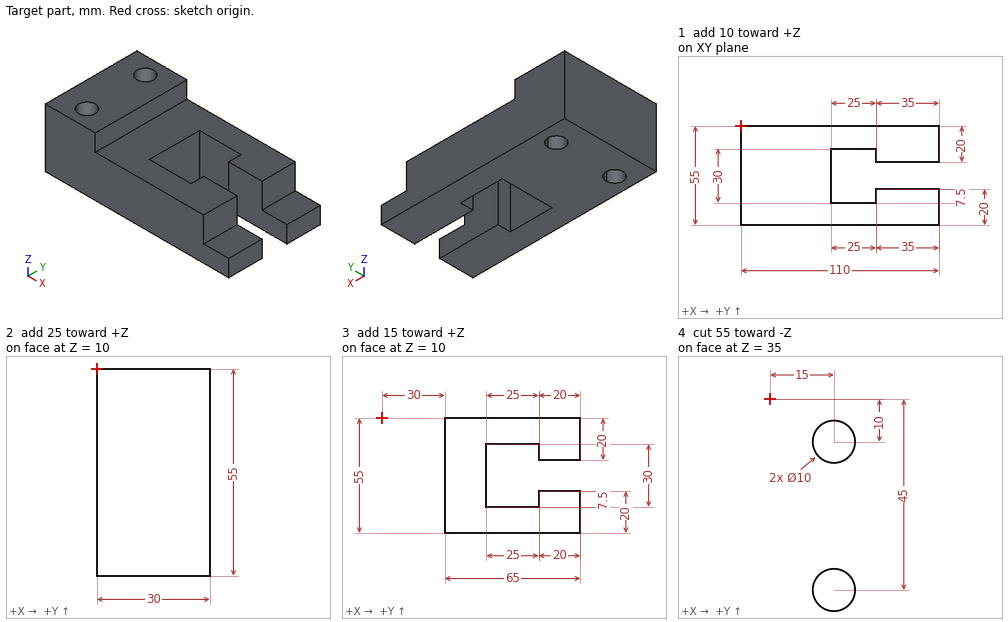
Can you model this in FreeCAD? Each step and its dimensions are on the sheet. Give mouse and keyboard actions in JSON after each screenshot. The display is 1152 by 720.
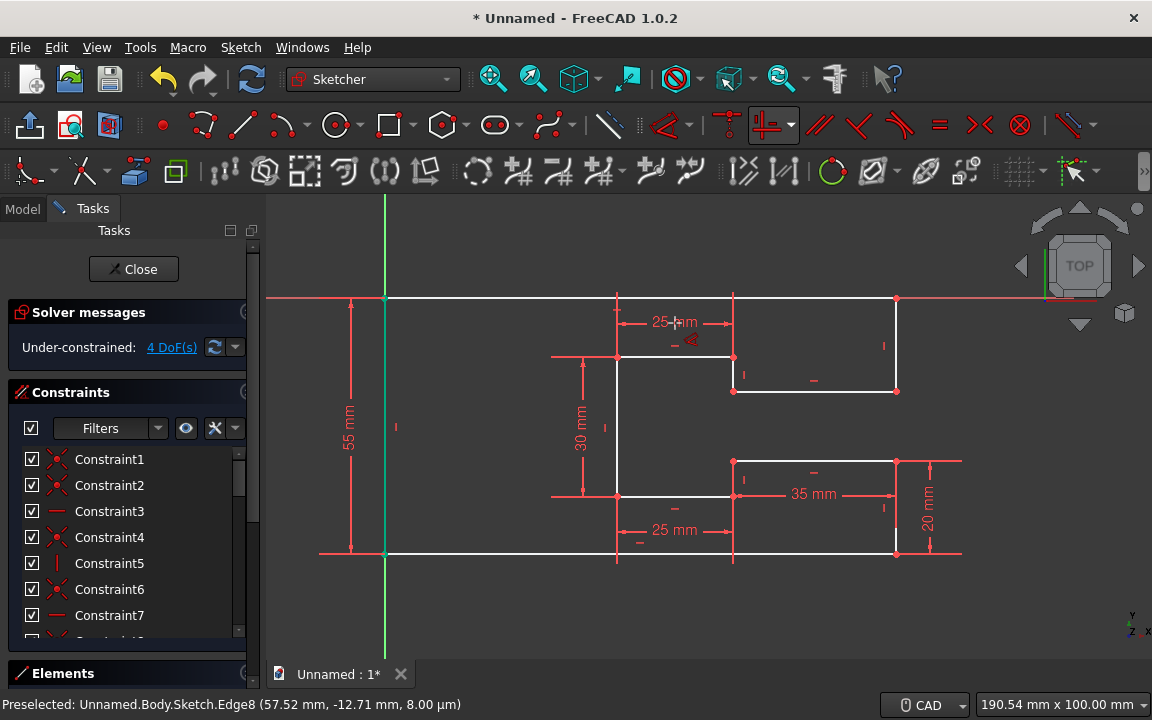
{"action": "left_click", "coordinate": [782, 392]}
{"action": "left_click", "coordinate": [815, 358]}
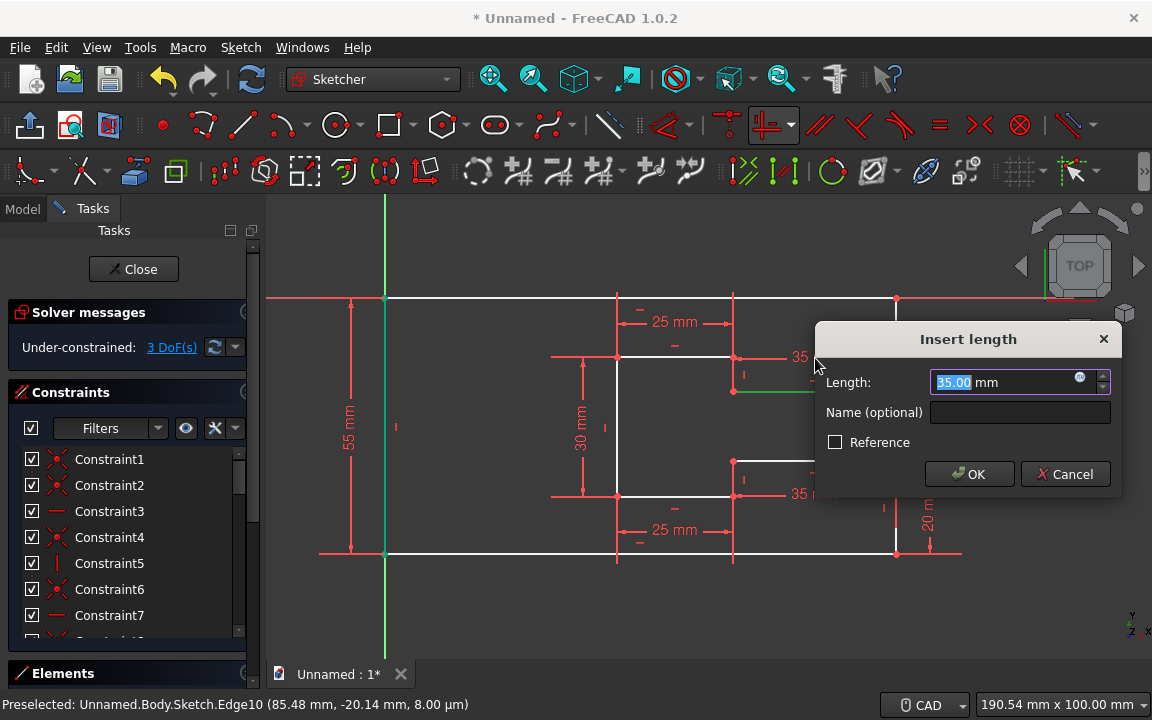
{"action": "type", "text": "35"}
{"action": "key", "text": "Return"}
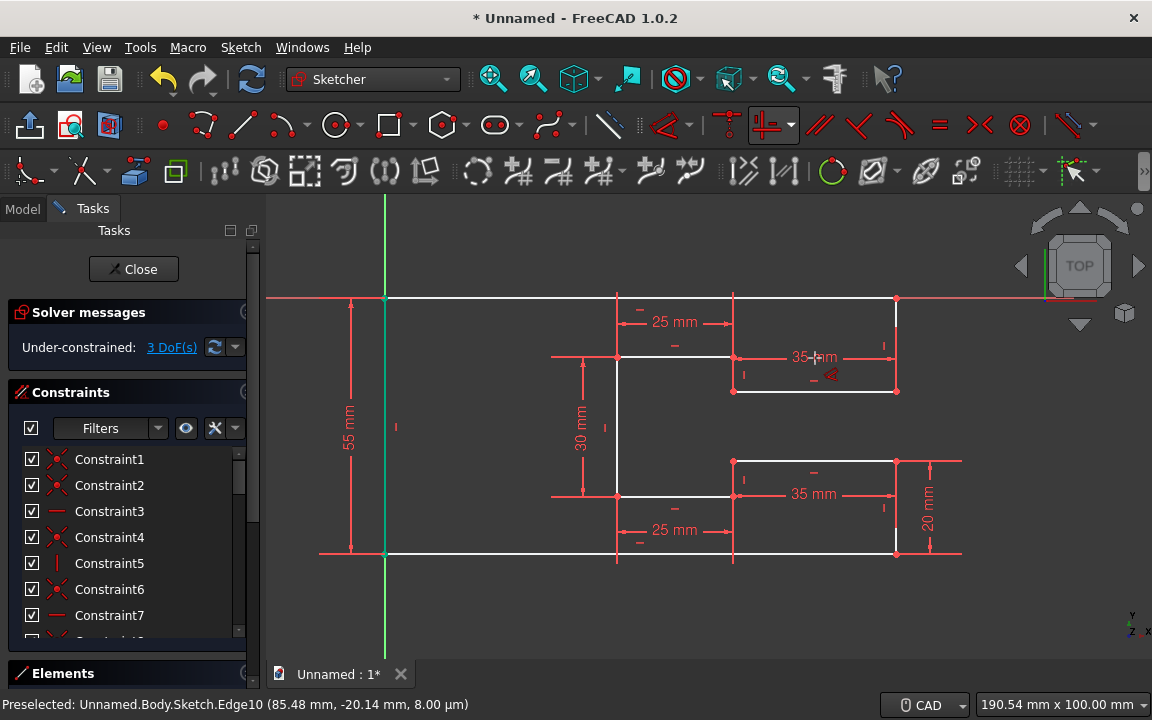
{"action": "left_click", "coordinate": [896, 364]}
{"action": "left_click", "coordinate": [930, 345]}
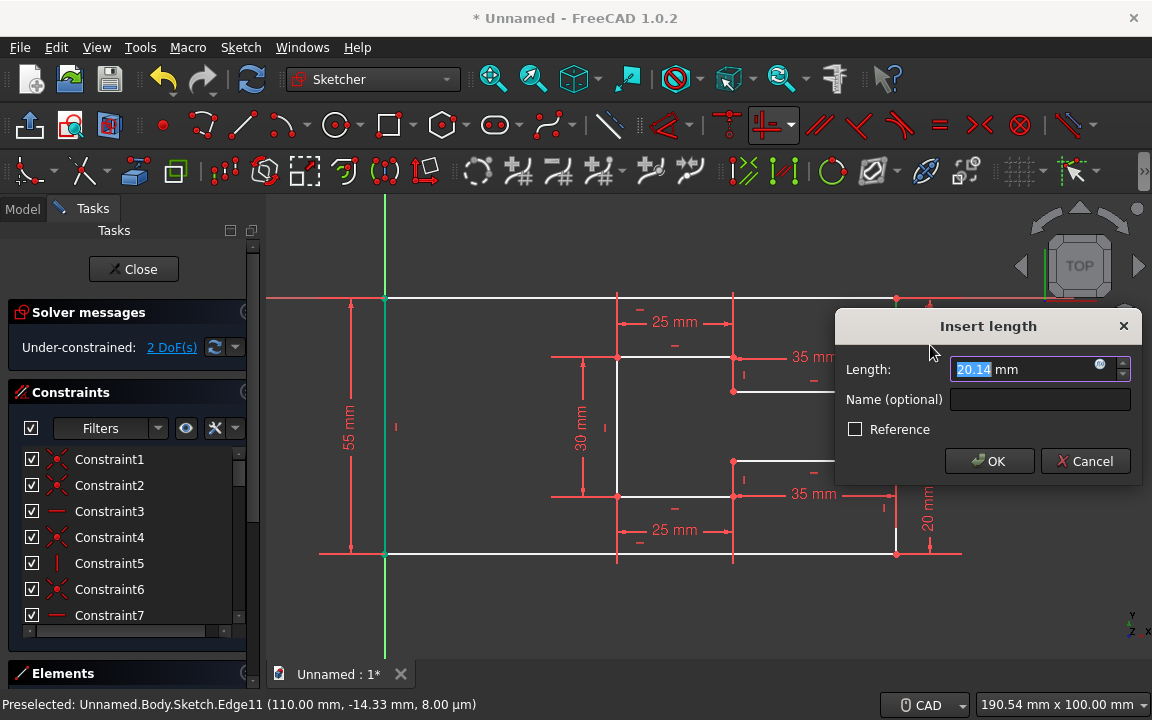
{"action": "type", "text": "20"}
{"action": "key", "text": "Return"}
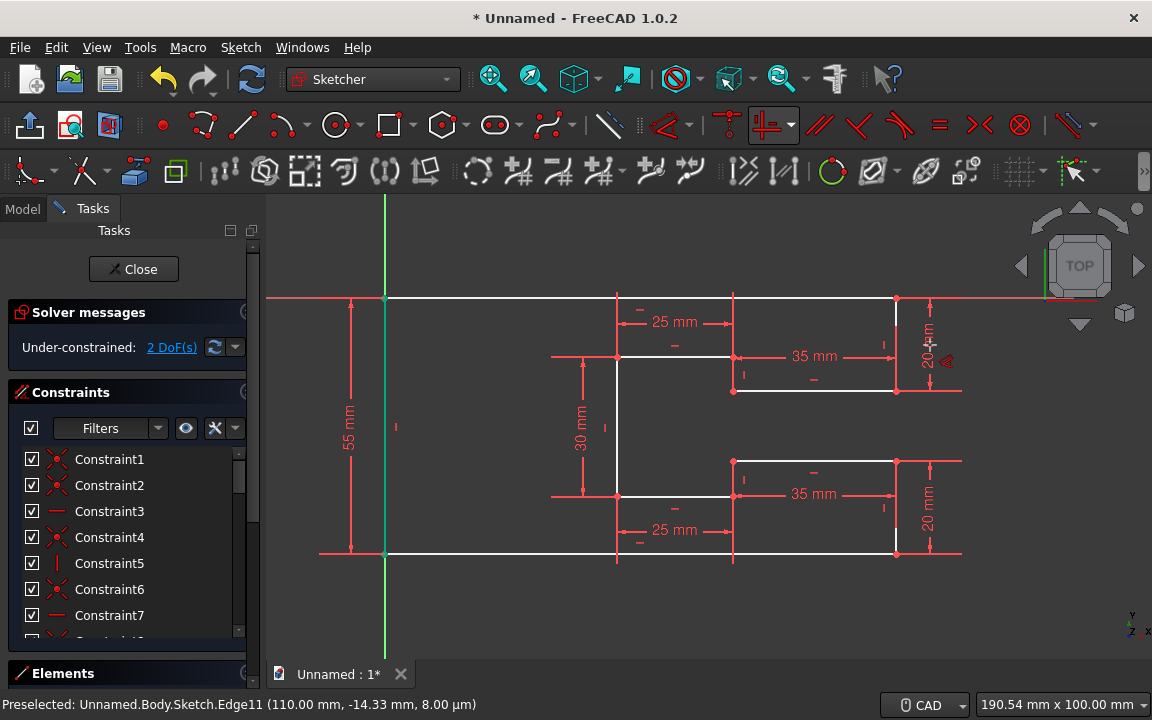
{"action": "left_click", "coordinate": [538, 554]}
{"action": "left_click", "coordinate": [640, 588]}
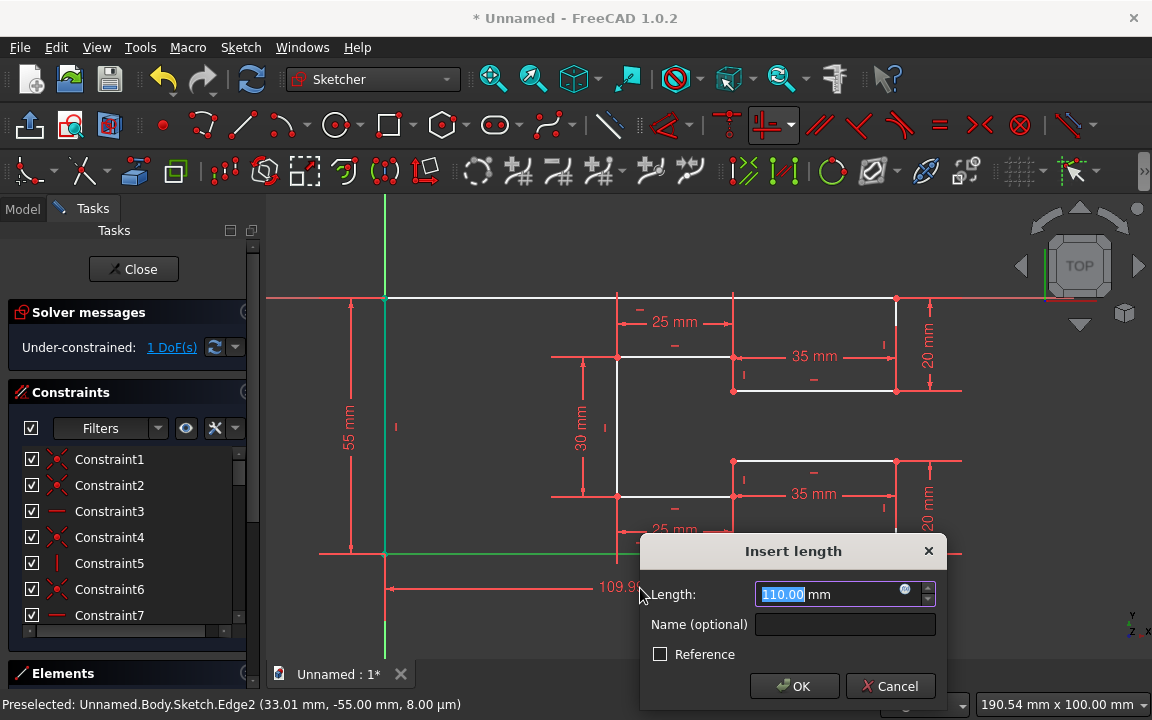
{"action": "type", "text": "110"}
{"action": "key", "text": "Return"}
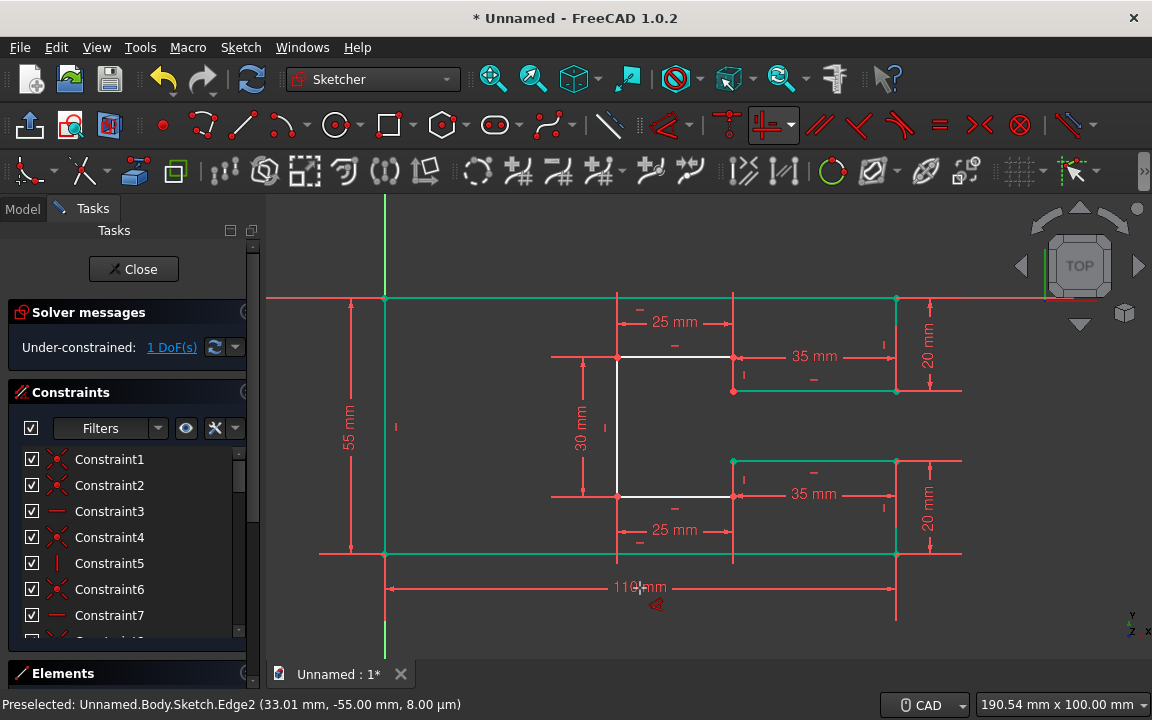
{"action": "scroll", "coordinate": [733, 472], "scroll_direction": "up", "scroll_amount": 2}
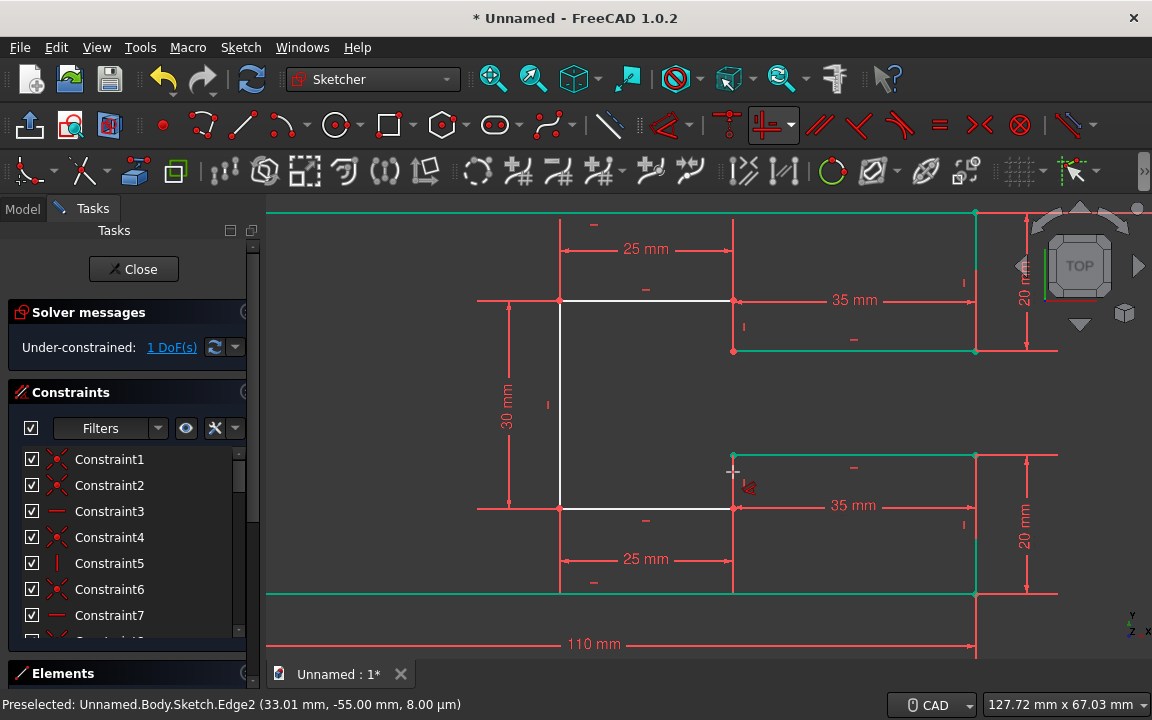
{"action": "left_click", "coordinate": [733, 471]}
{"action": "left_click", "coordinate": [767, 482]}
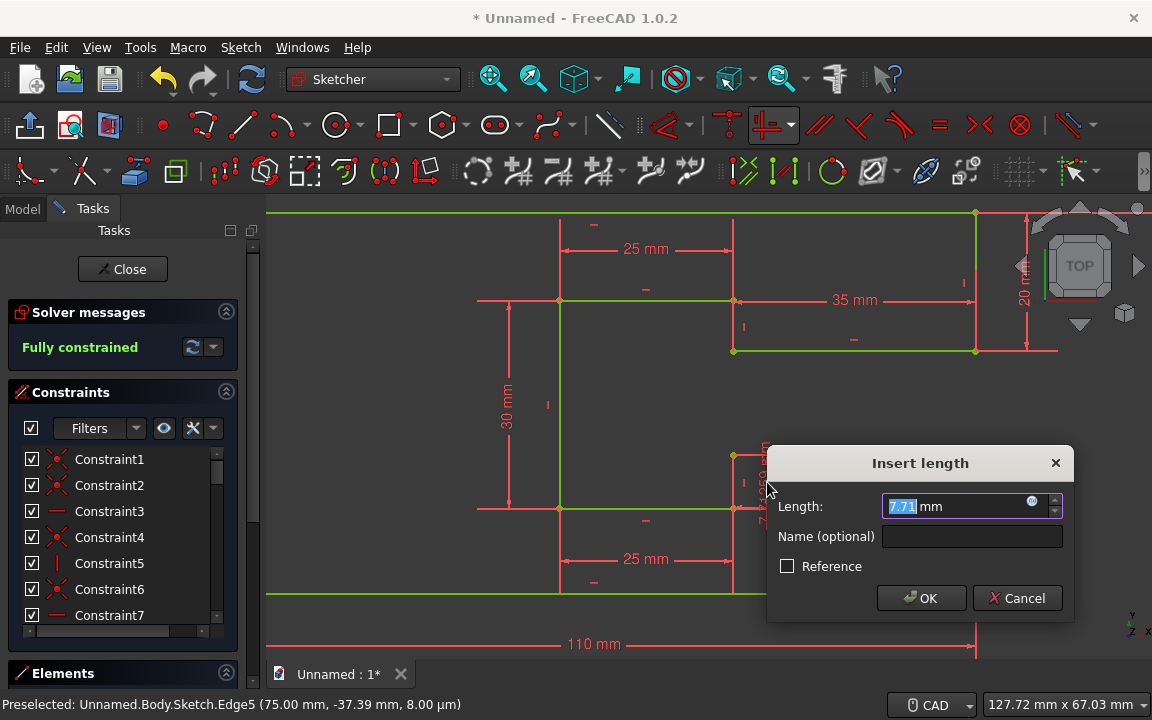
{"action": "type", "text": "7.5"}
{"action": "key", "text": "Return"}
{"action": "key", "text": "Escape"}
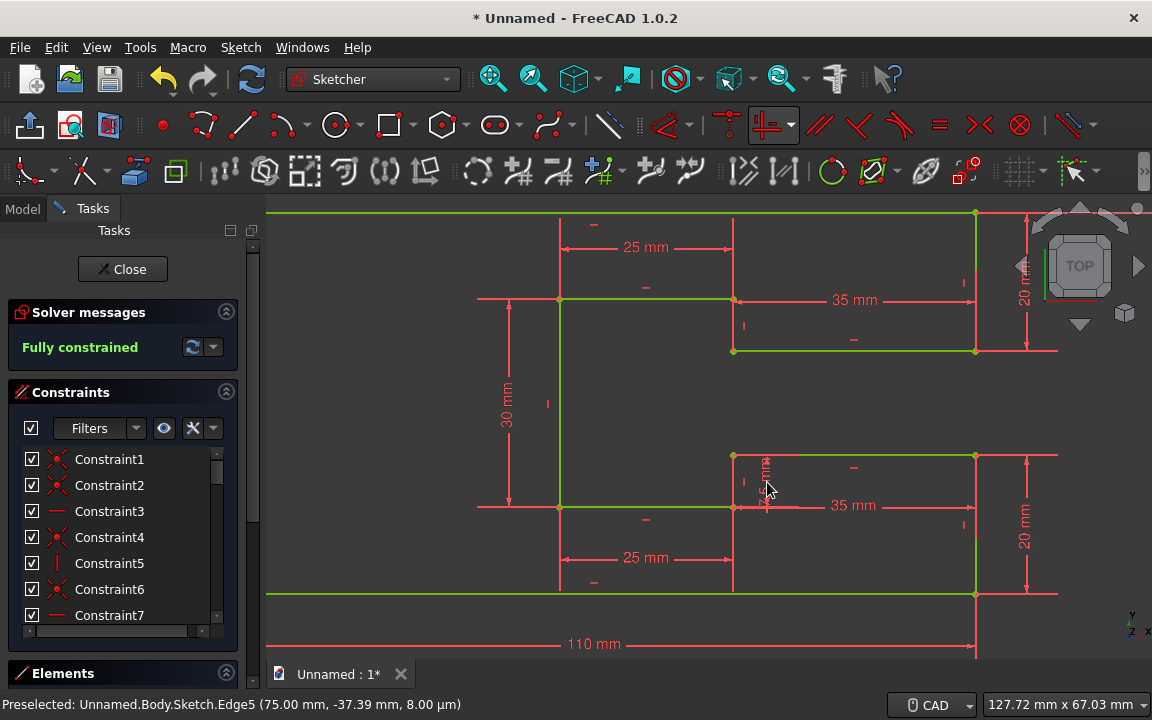
{"action": "left_click", "coordinate": [123, 269]}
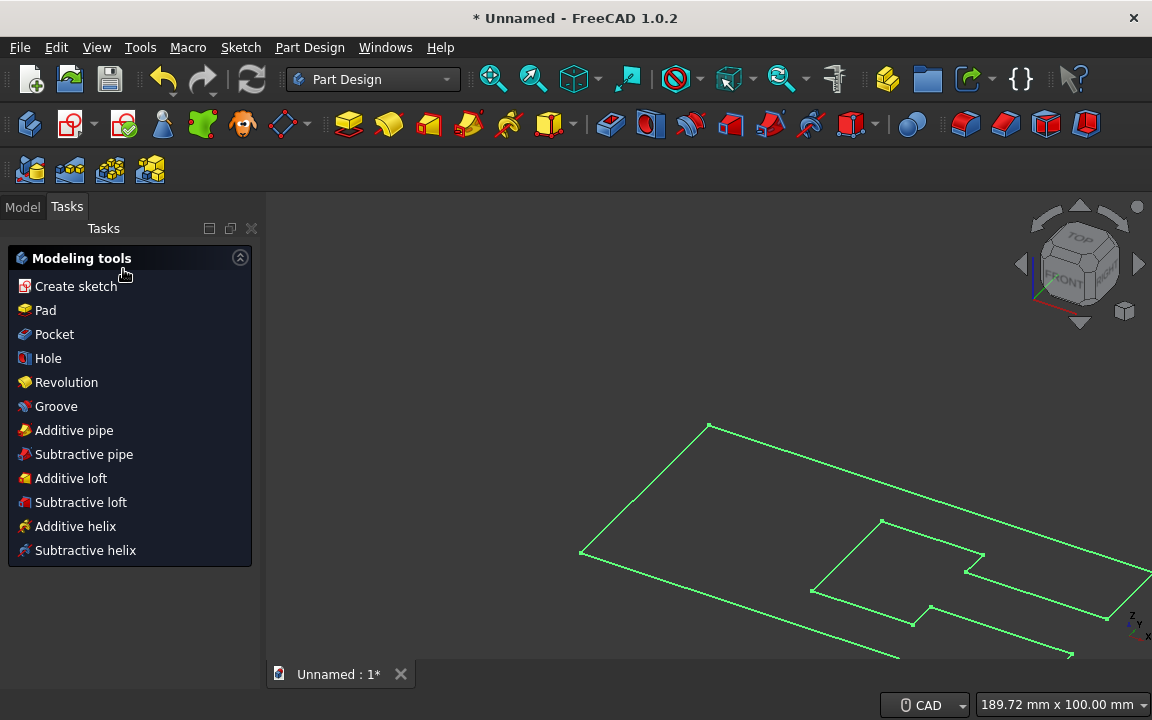
{"action": "left_click", "coordinate": [350, 124]}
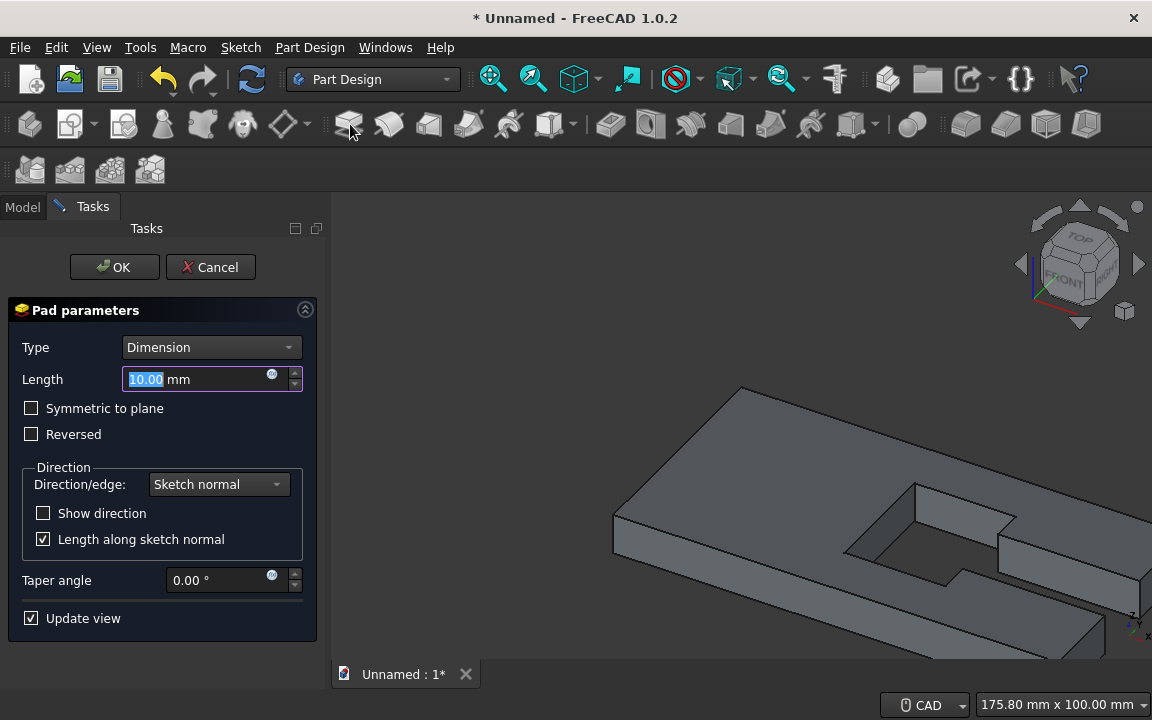
{"action": "type", "text": "10"}
{"action": "key", "text": "Tab"}